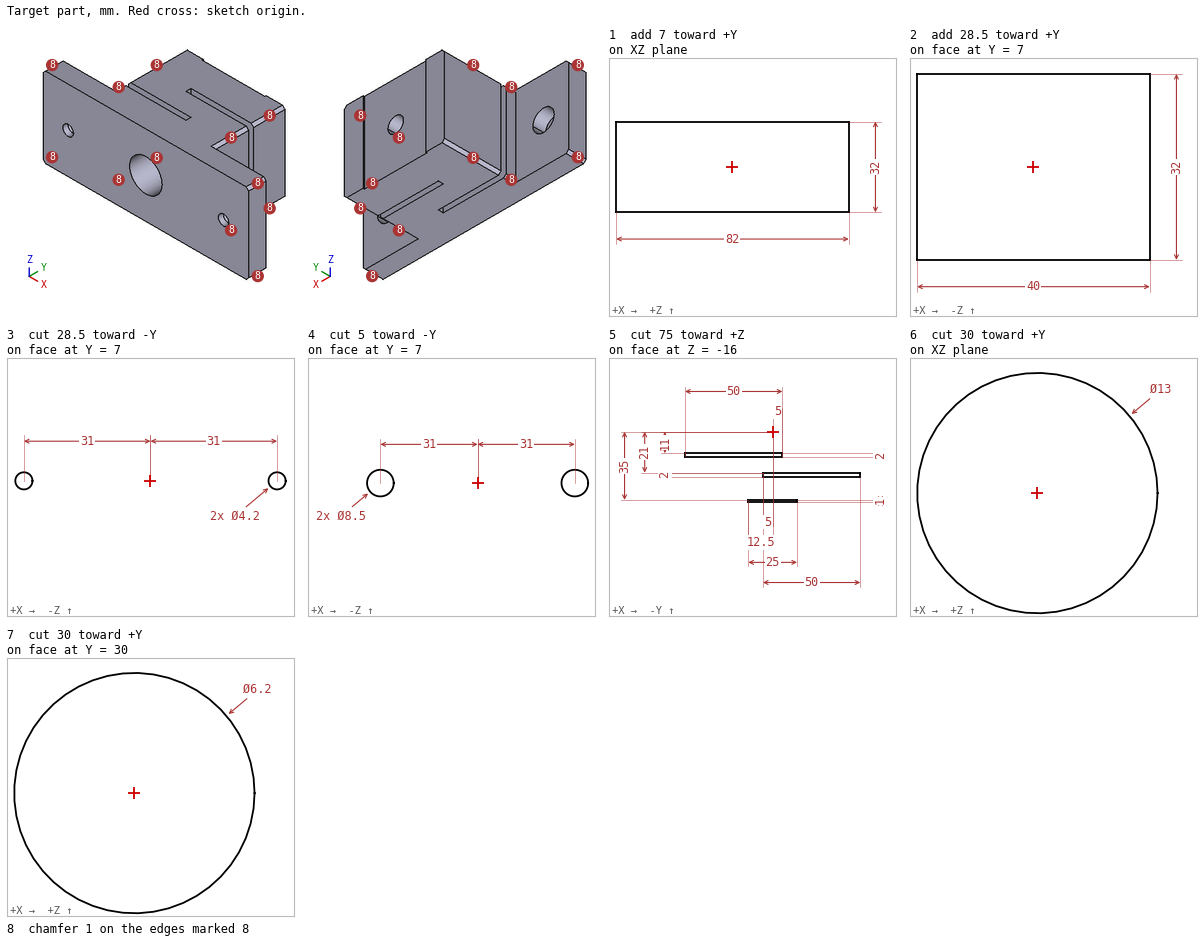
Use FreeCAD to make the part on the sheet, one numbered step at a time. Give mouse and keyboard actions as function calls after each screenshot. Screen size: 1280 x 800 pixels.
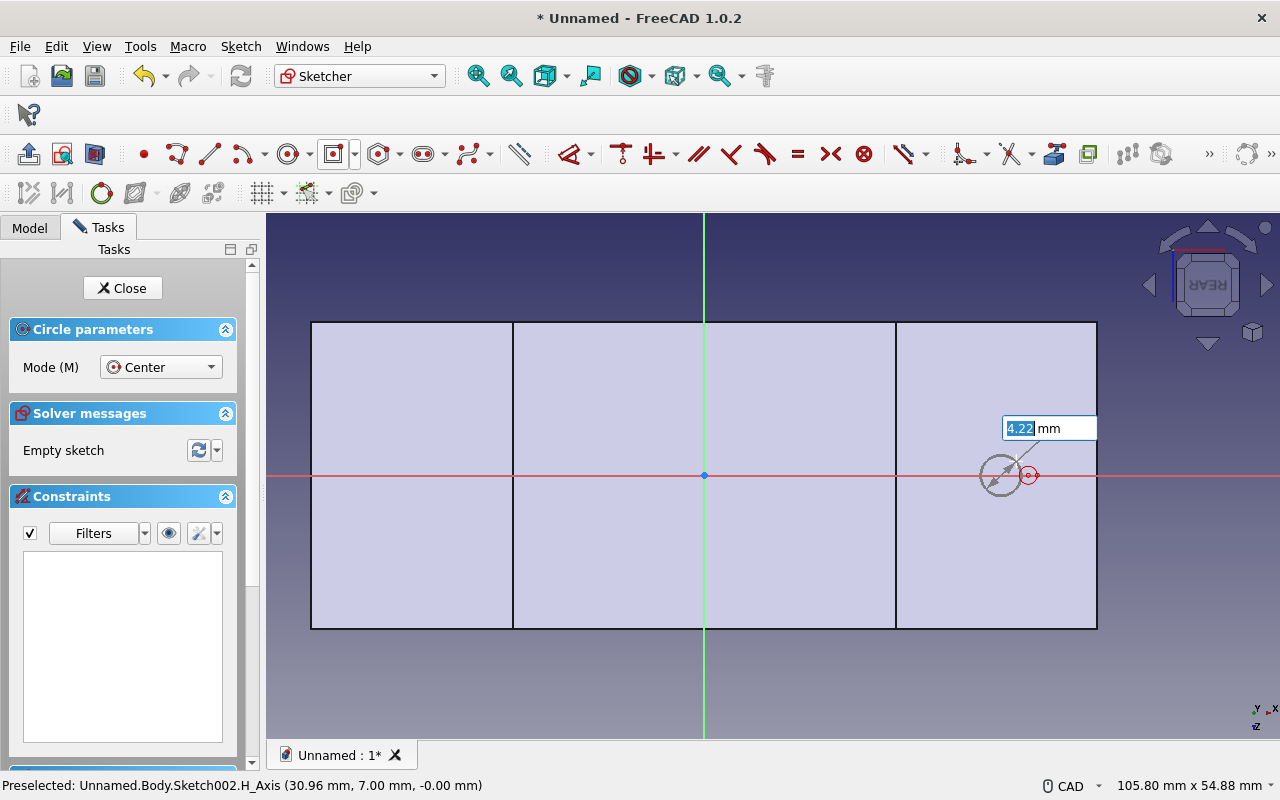
text(4.2)
key(Return)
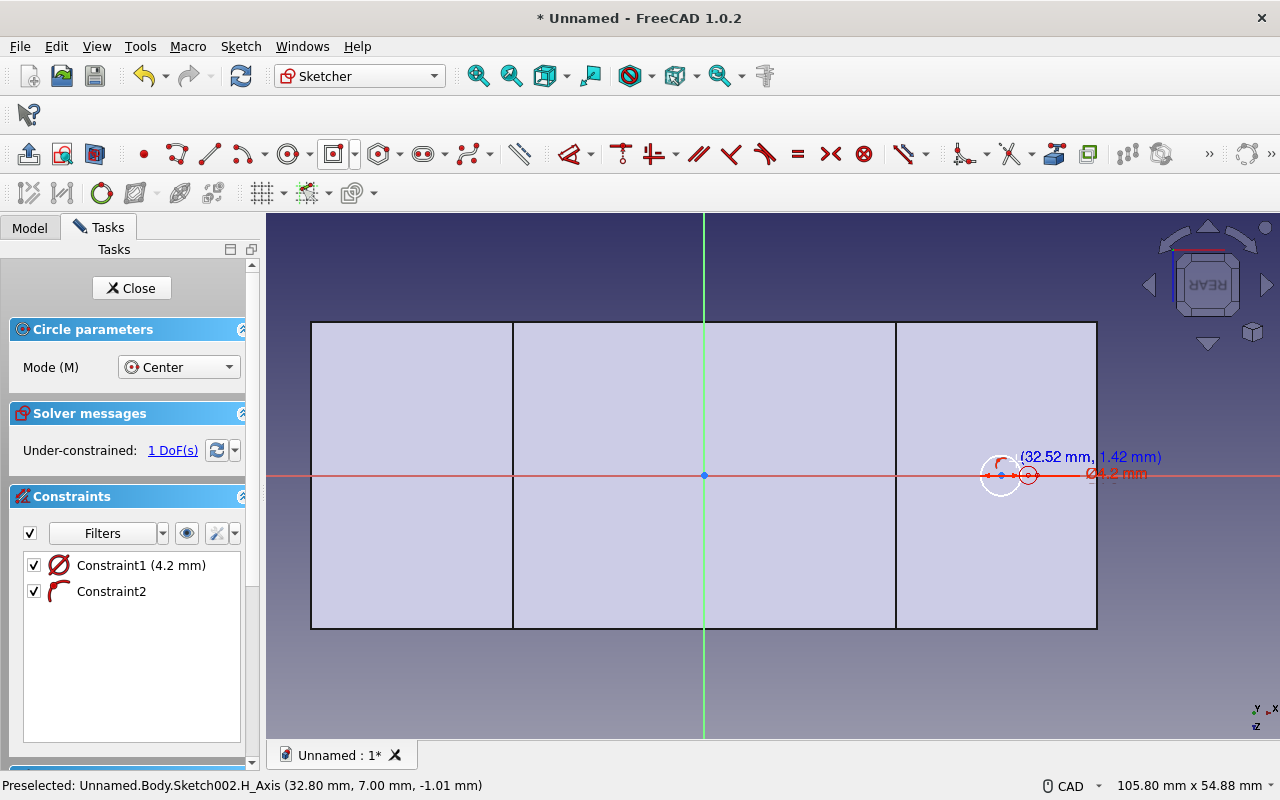
click(407, 476)
move(421, 461)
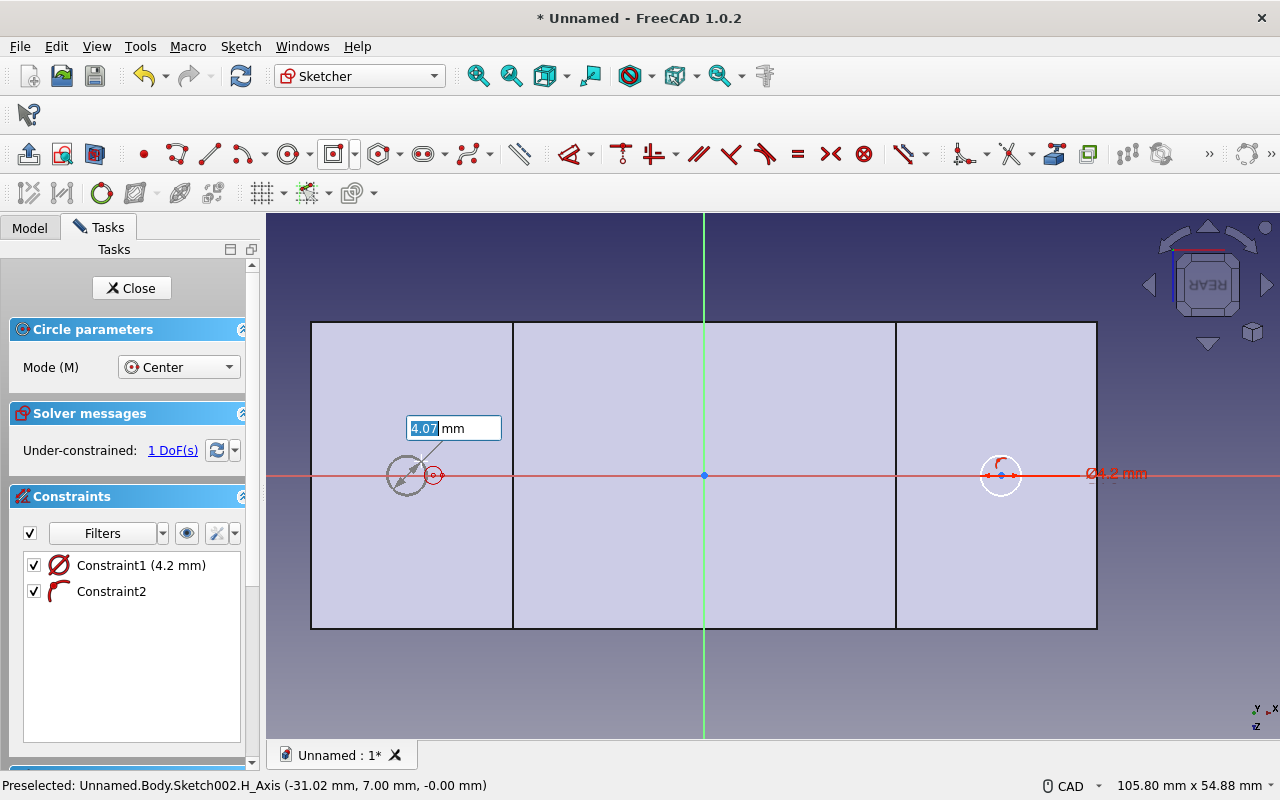
text(4.2)
key(Return)
key(Escape)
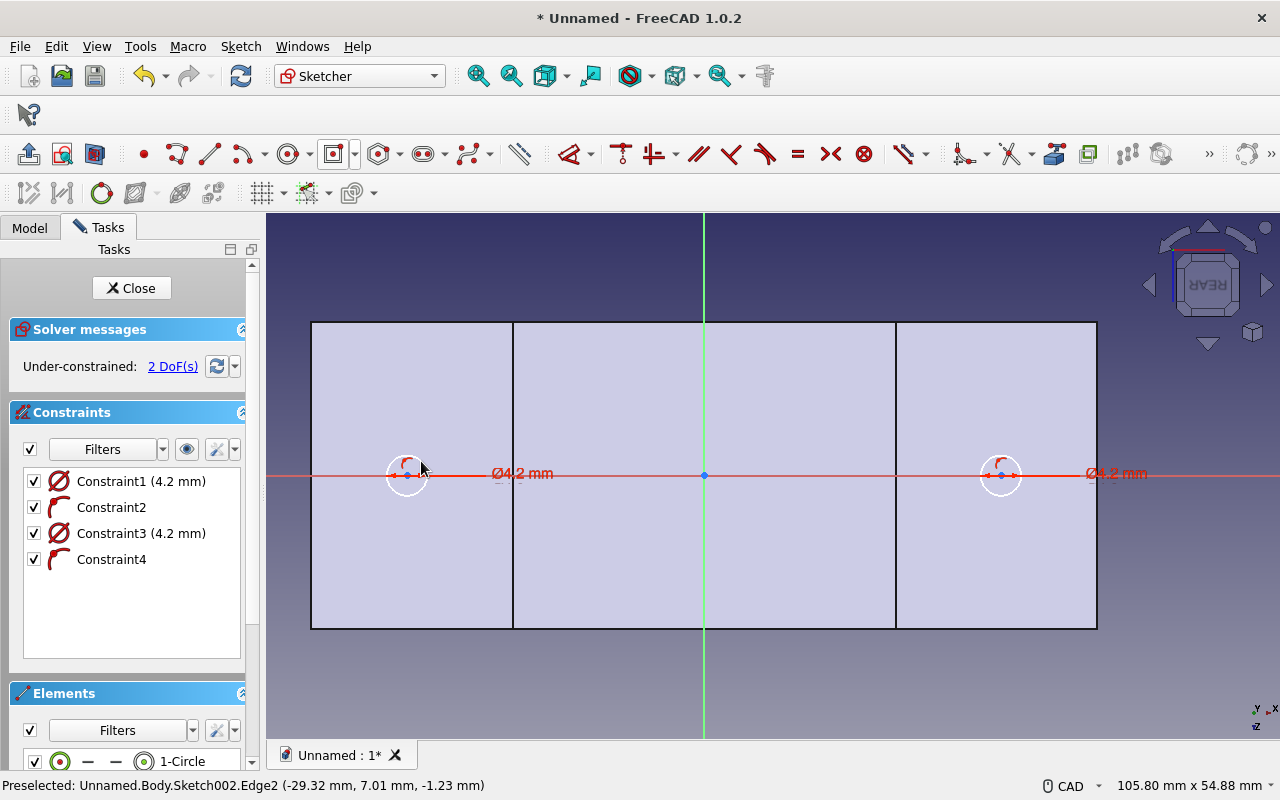
key(d)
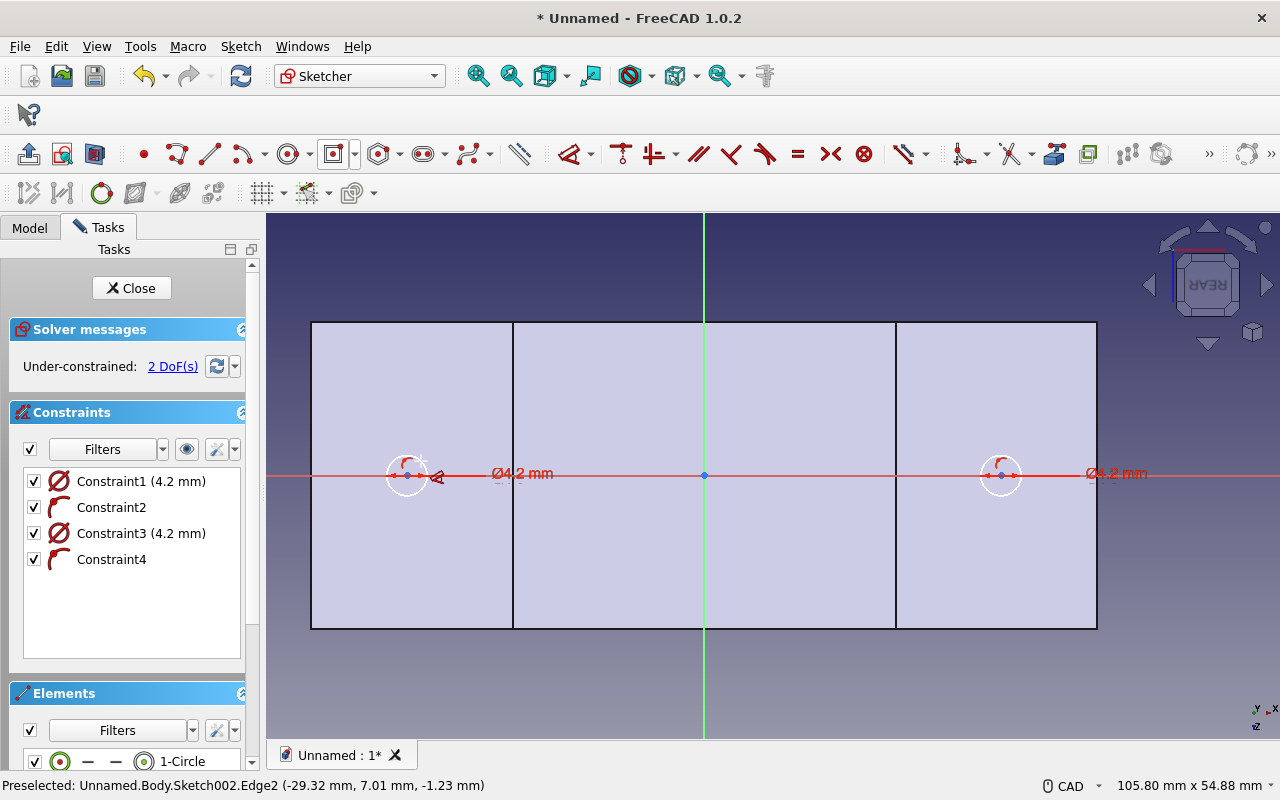
click(1001, 476)
click(853, 510)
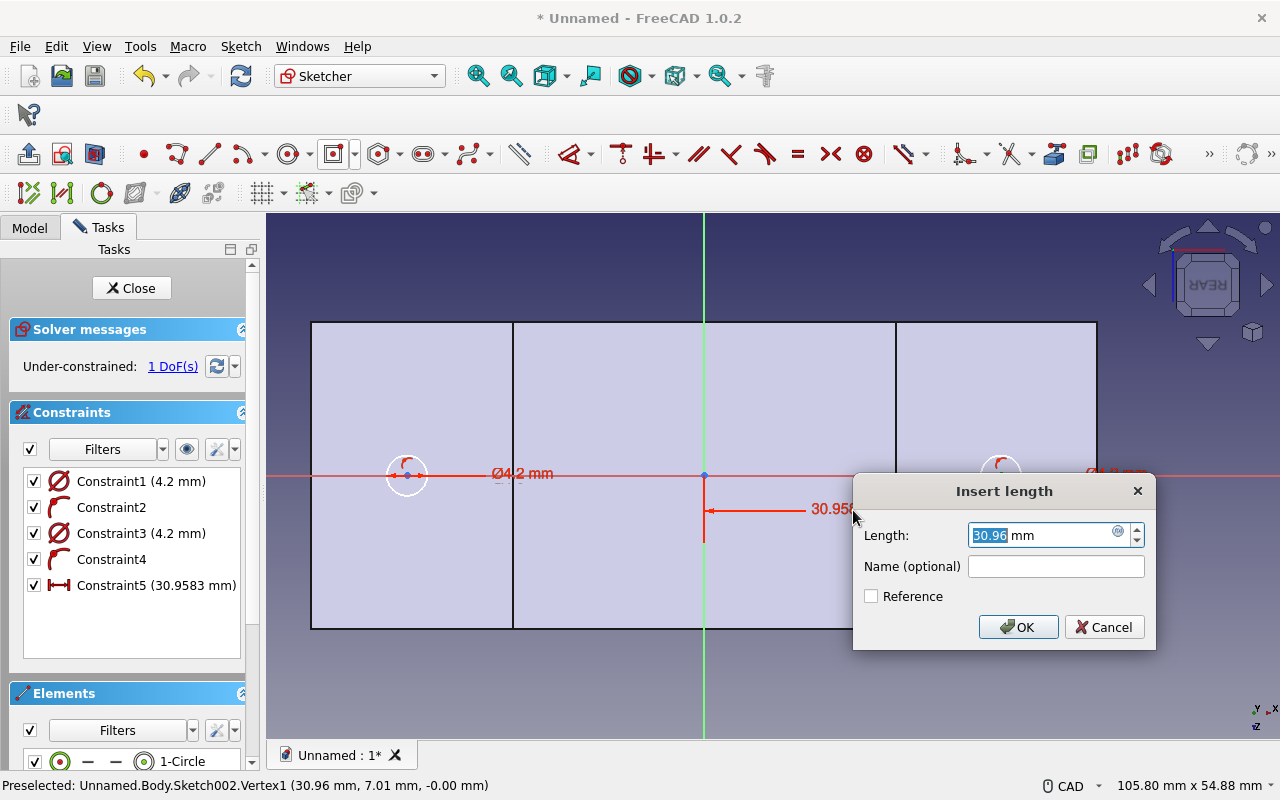
text(31)
key(Return)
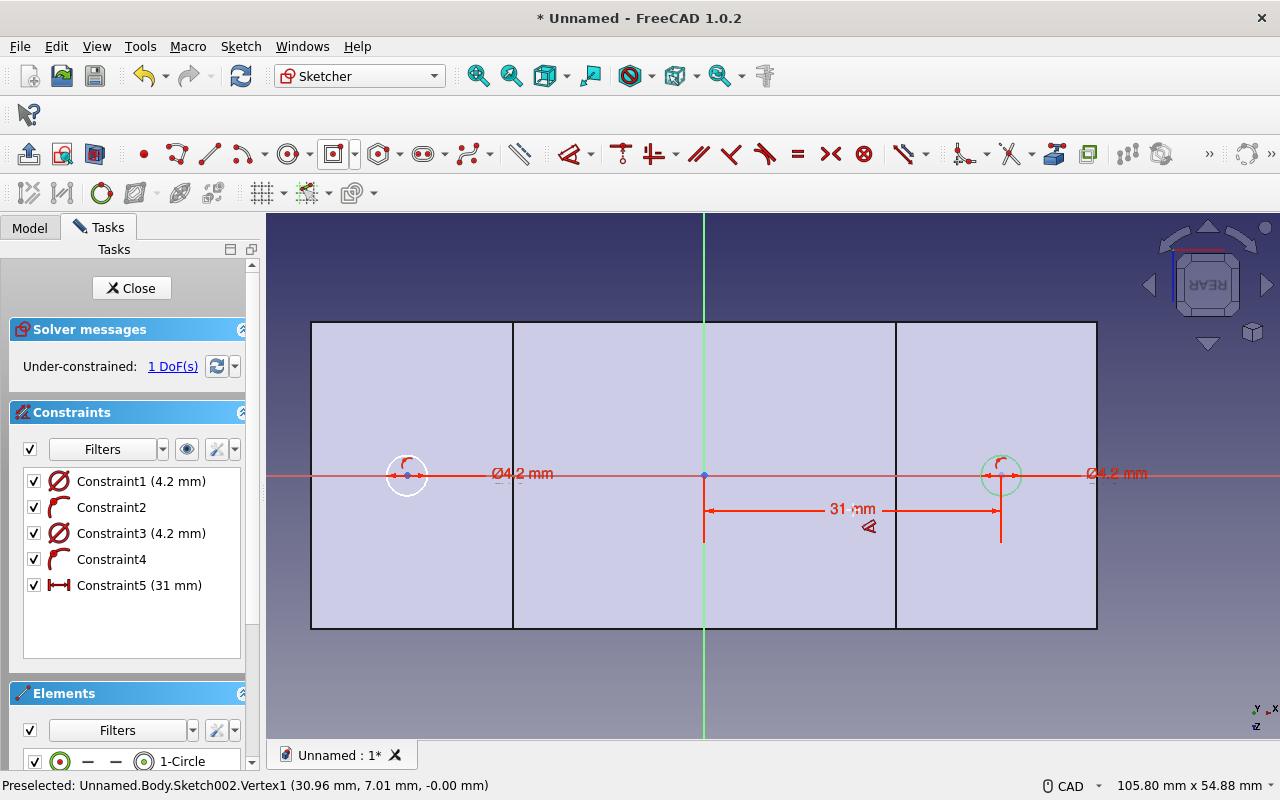
click(407, 476)
click(556, 510)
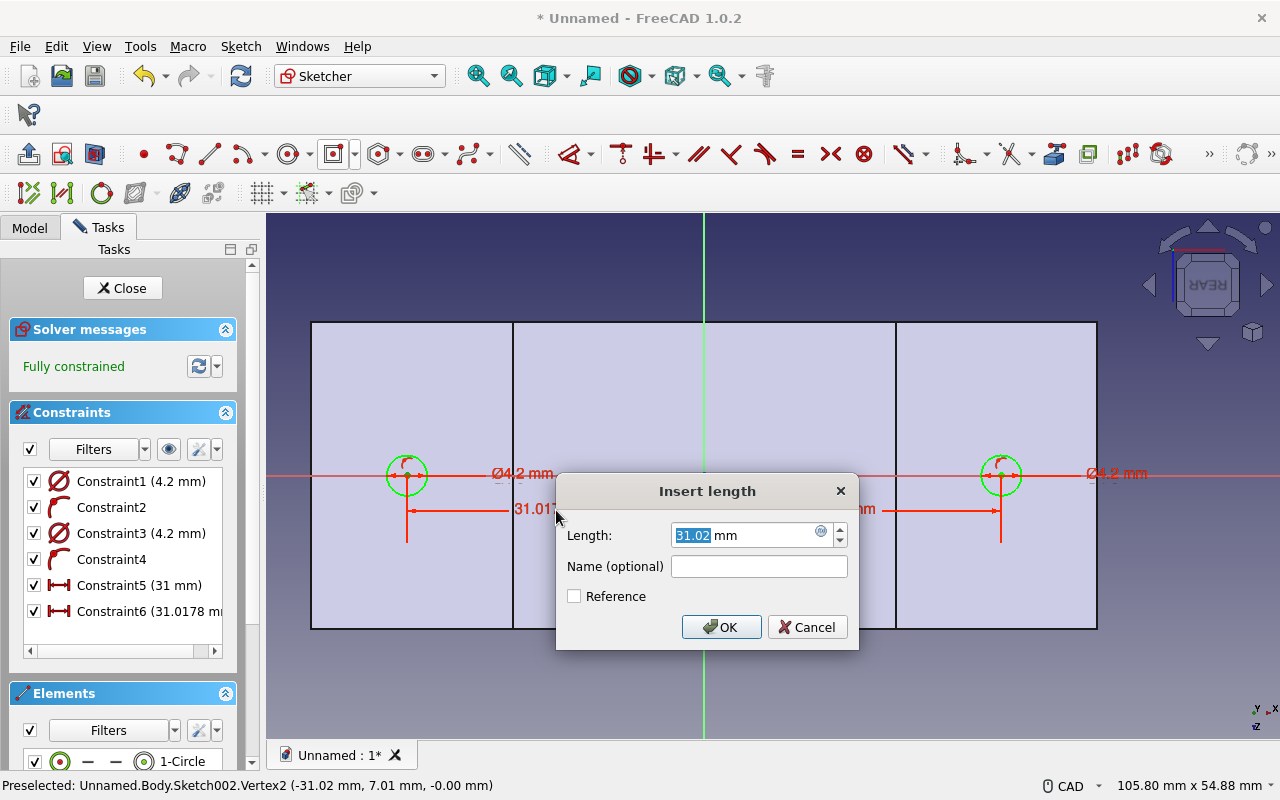
text(31)
key(Return)
key(Escape)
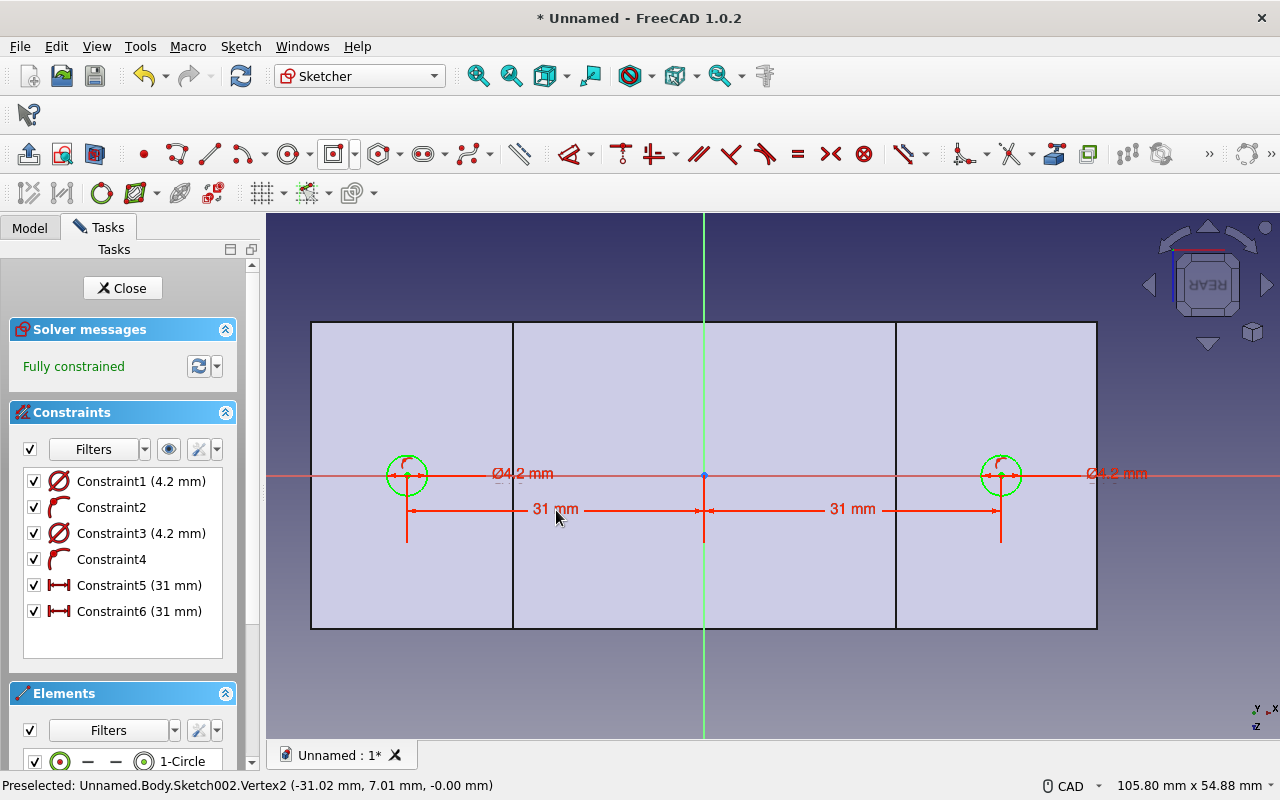
click(123, 288)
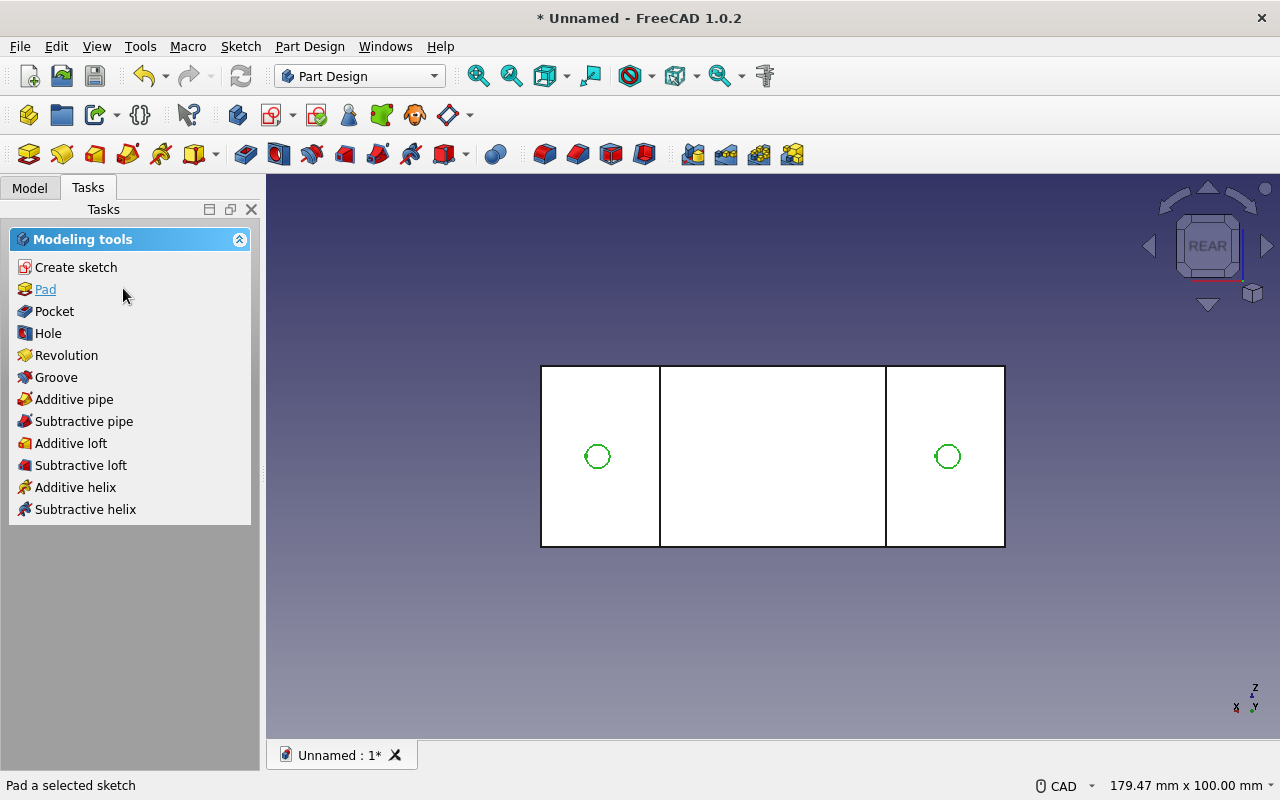
click(246, 154)